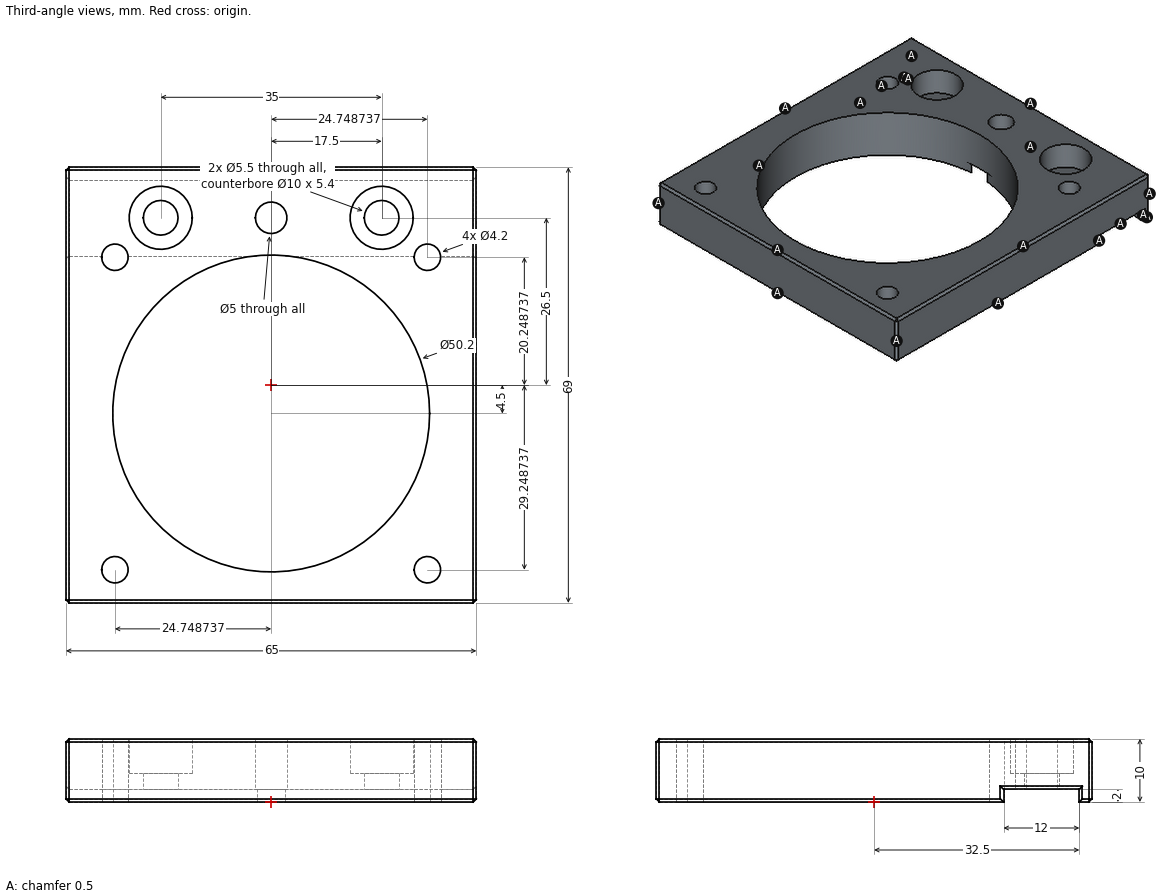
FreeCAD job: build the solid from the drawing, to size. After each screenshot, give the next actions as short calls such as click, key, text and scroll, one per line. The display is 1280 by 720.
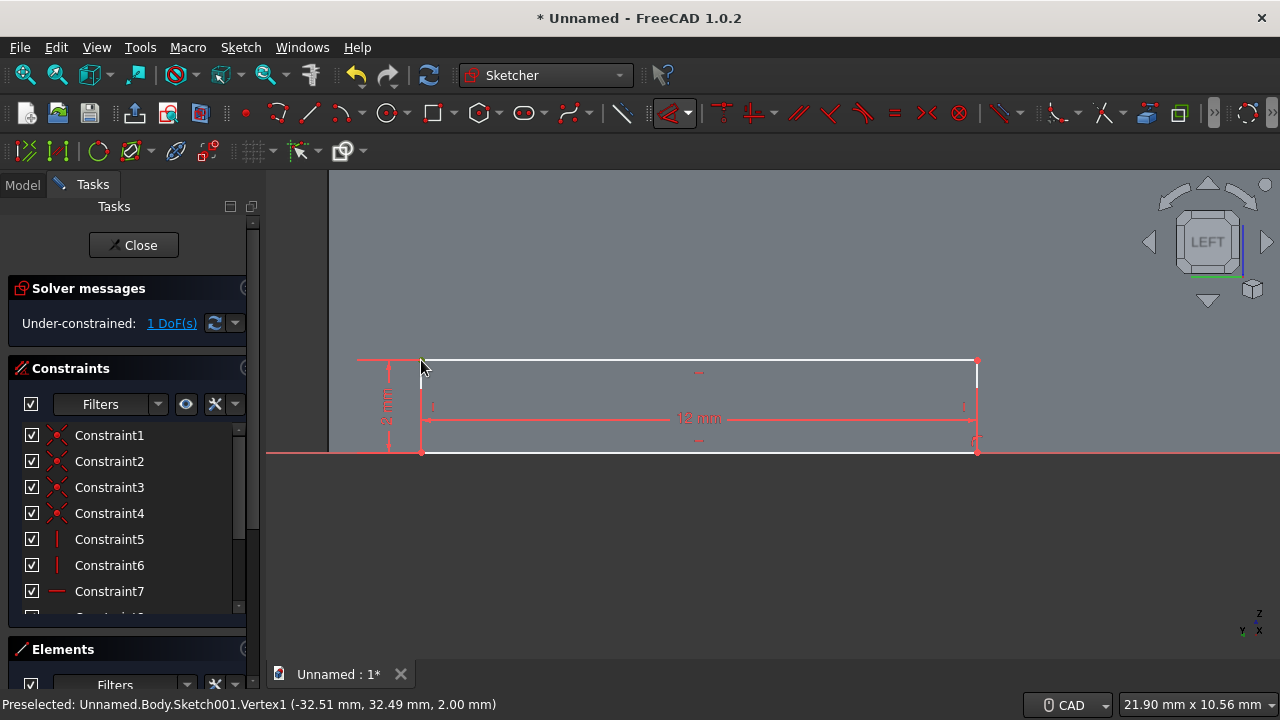
key(l)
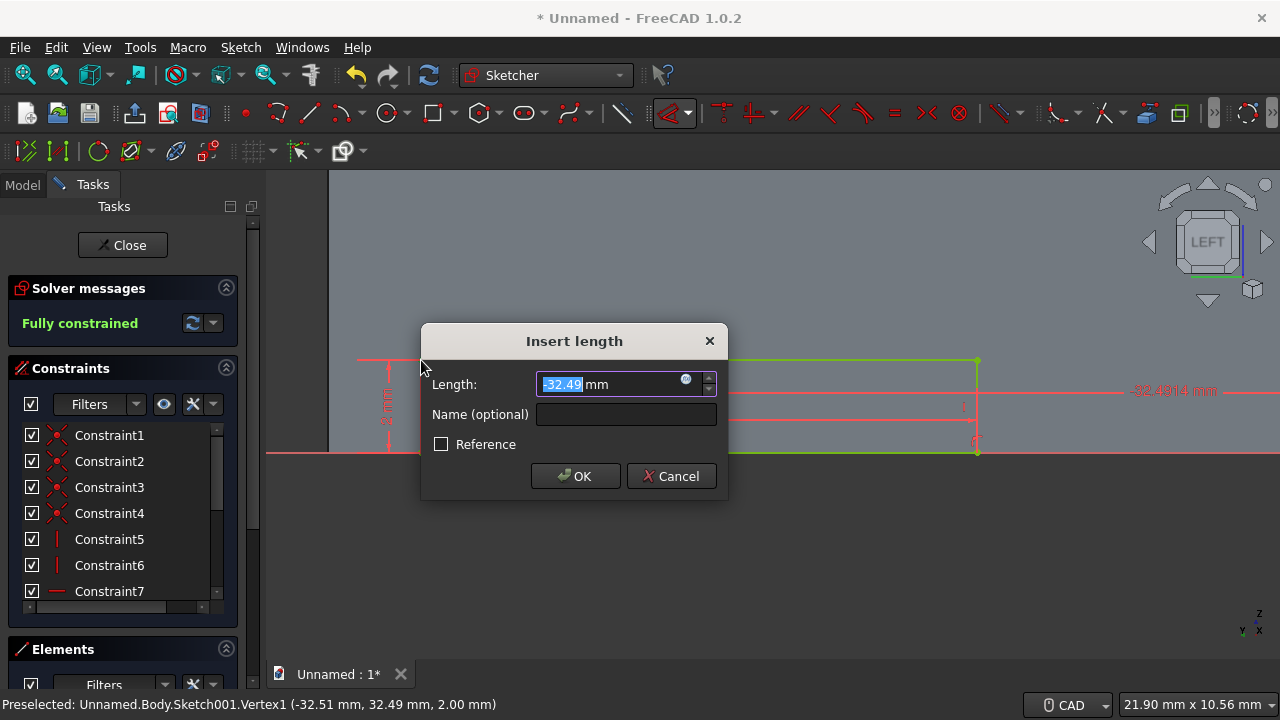
text(-32.5)
key(Return)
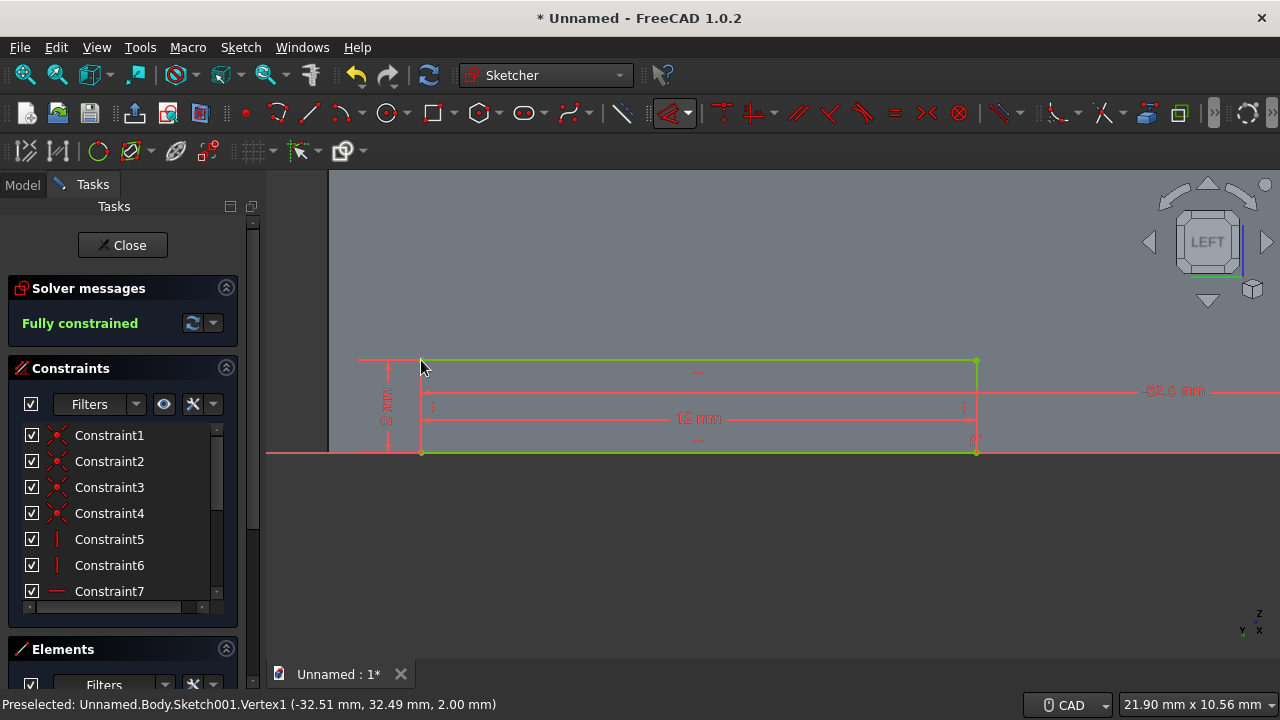
click(123, 245)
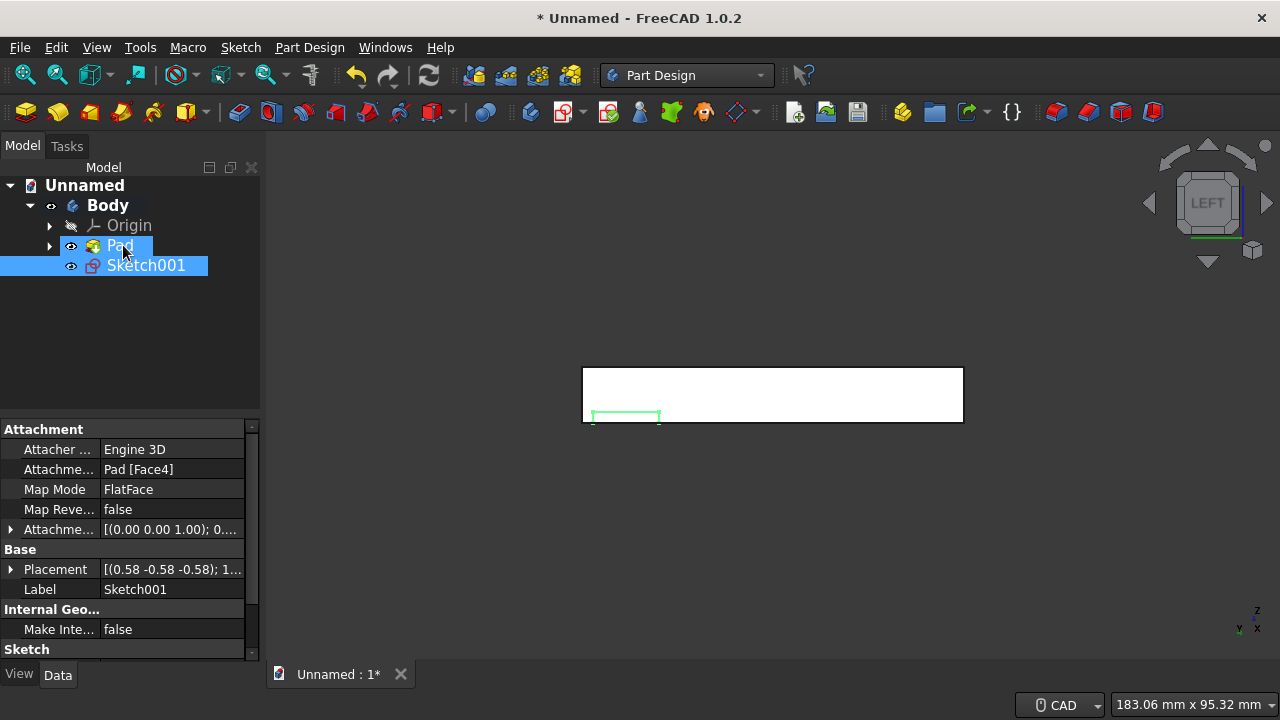
click(240, 112)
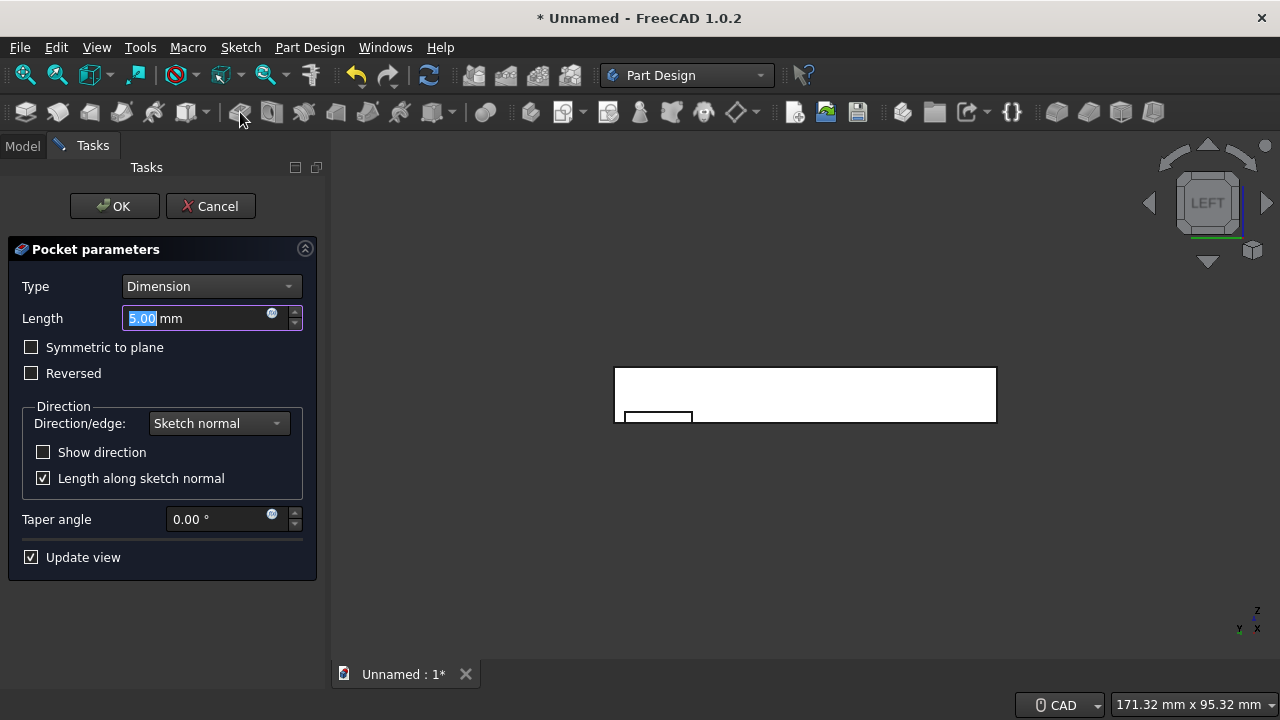
click(212, 286)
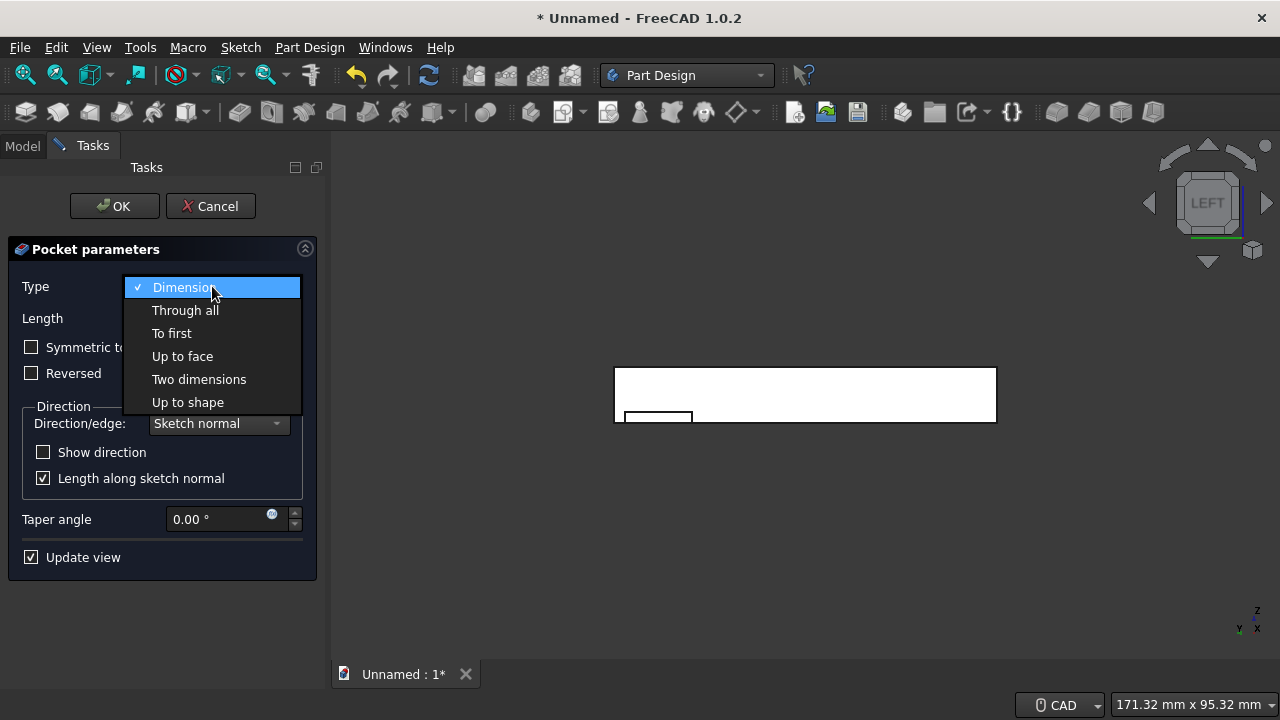
click(212, 310)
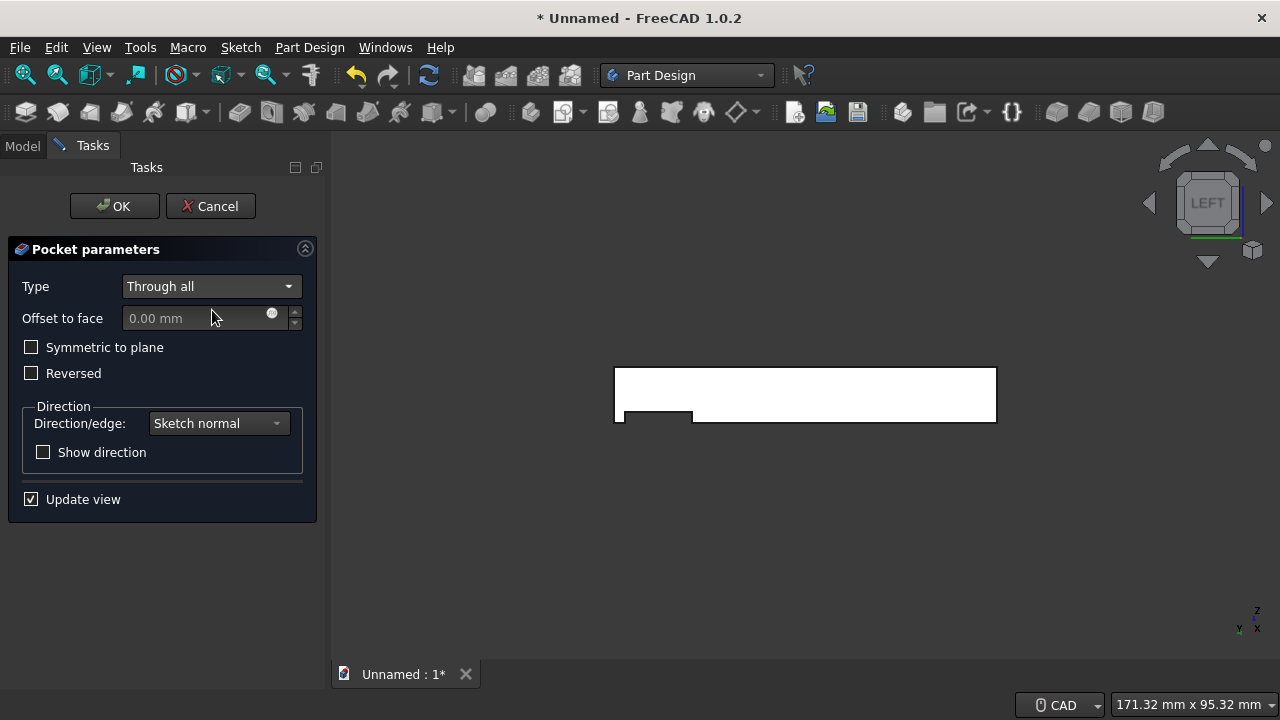
click(115, 206)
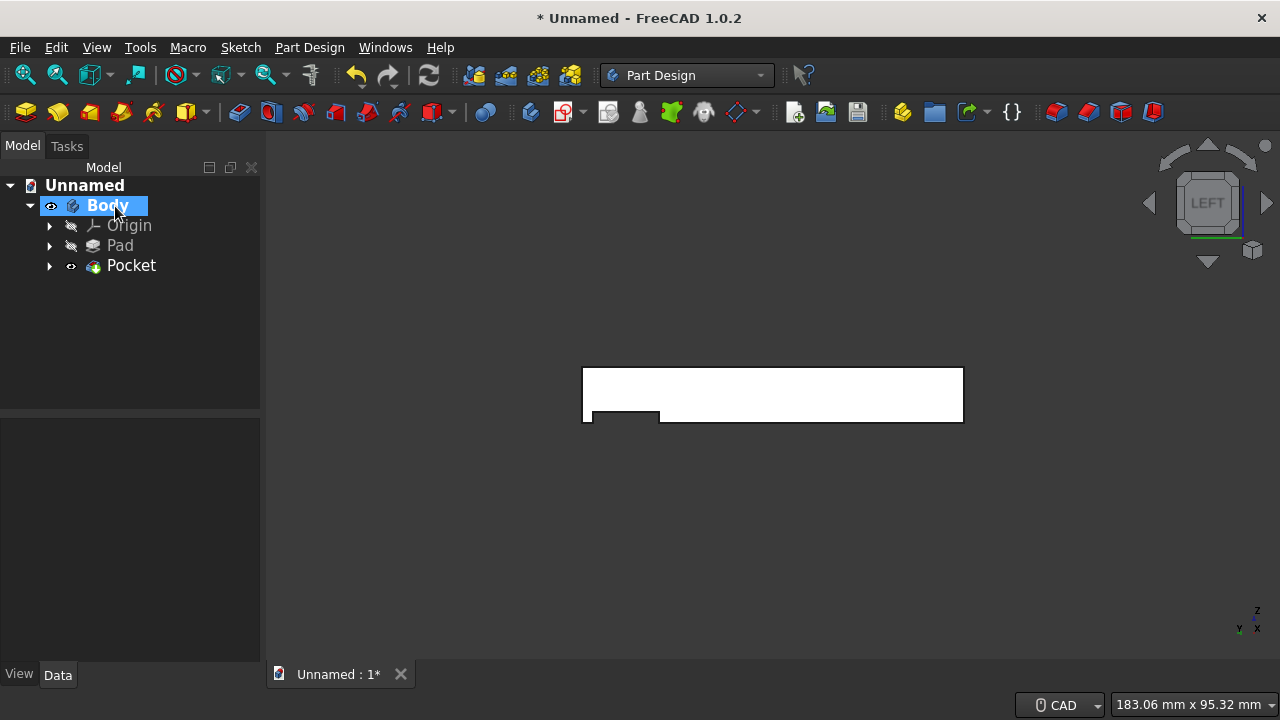
click(26, 76)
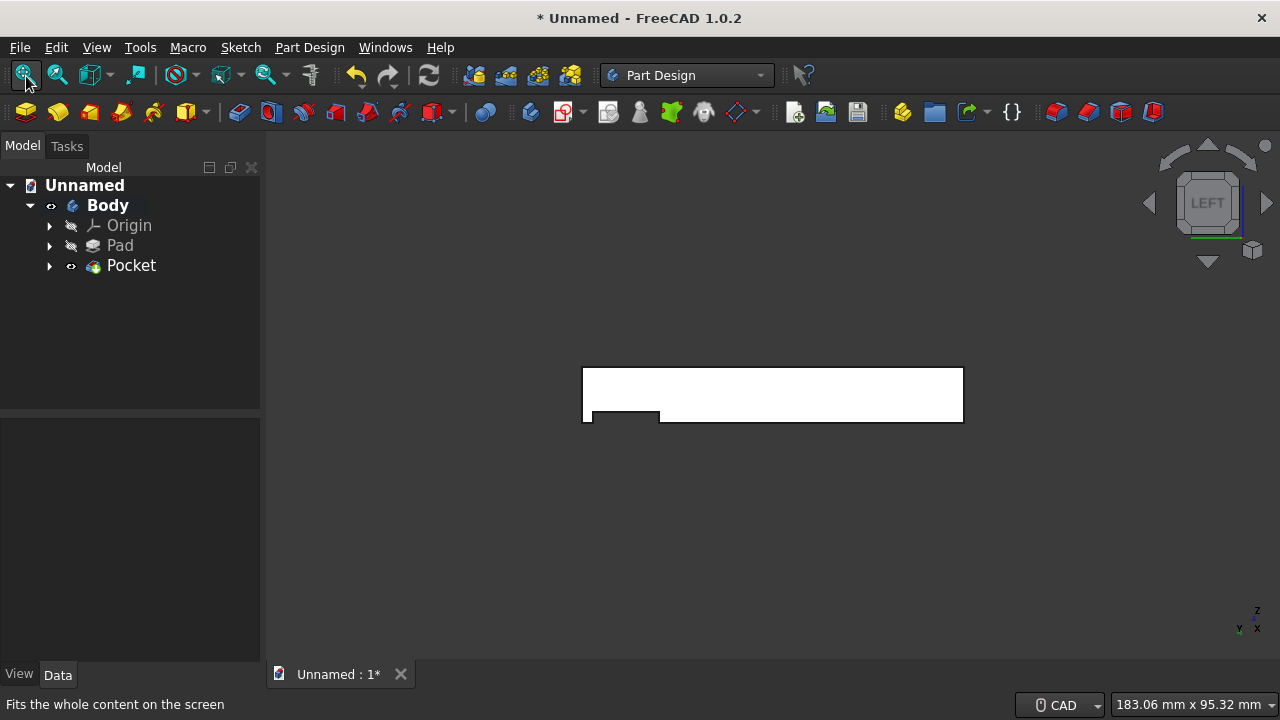
key(0)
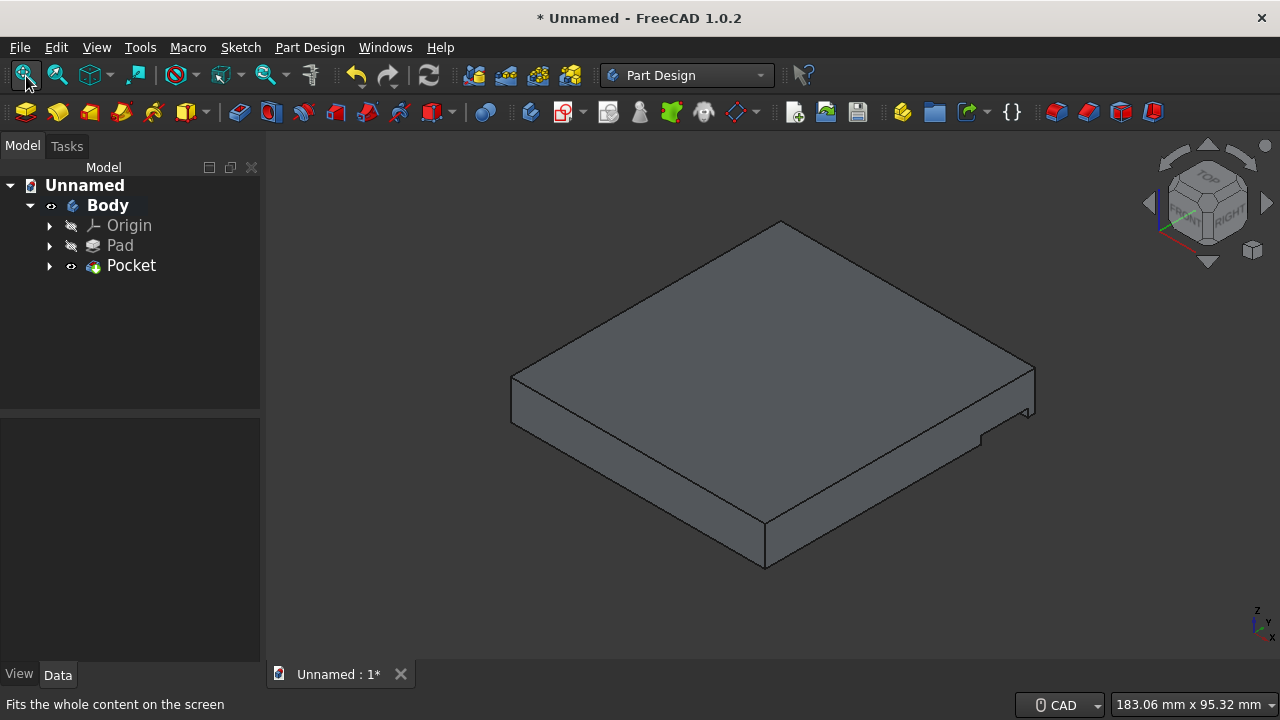
click(773, 371)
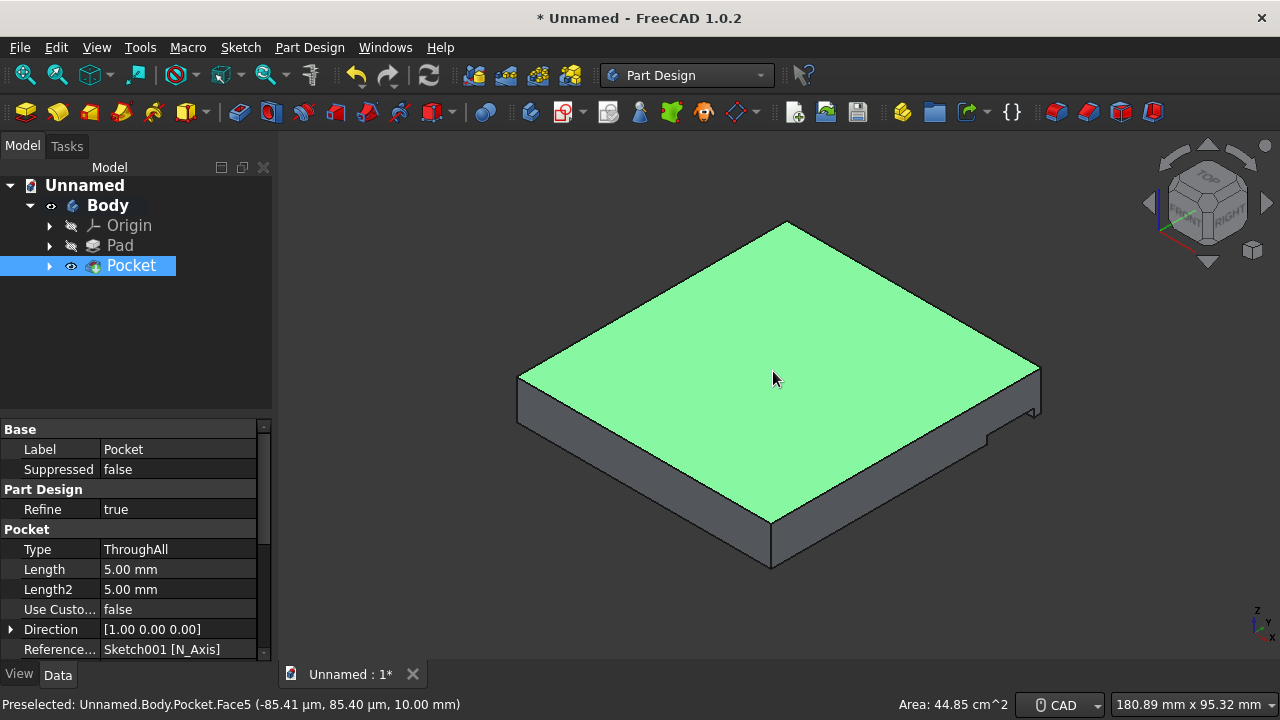
click(564, 112)